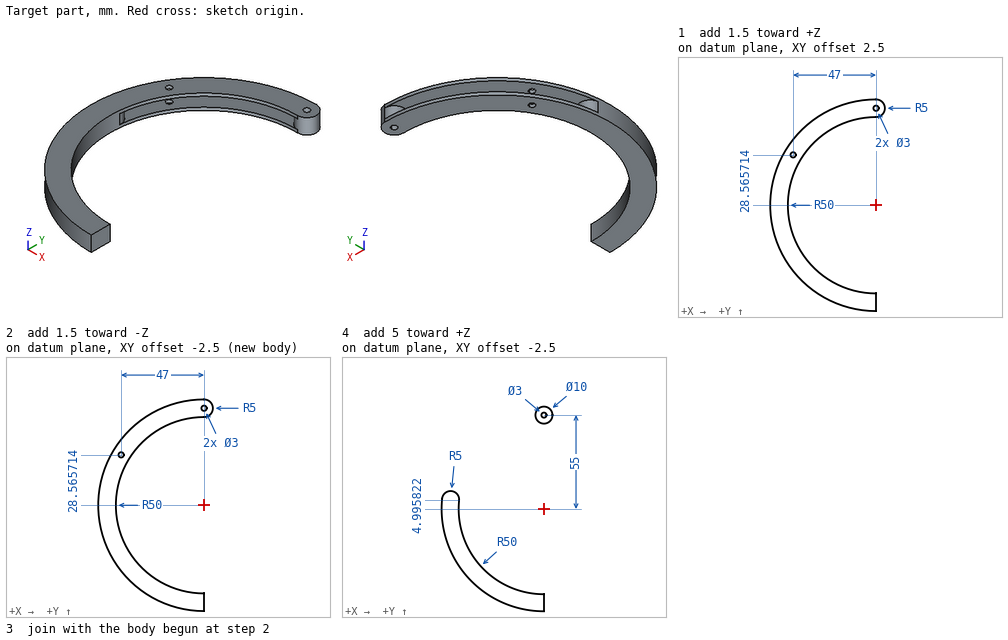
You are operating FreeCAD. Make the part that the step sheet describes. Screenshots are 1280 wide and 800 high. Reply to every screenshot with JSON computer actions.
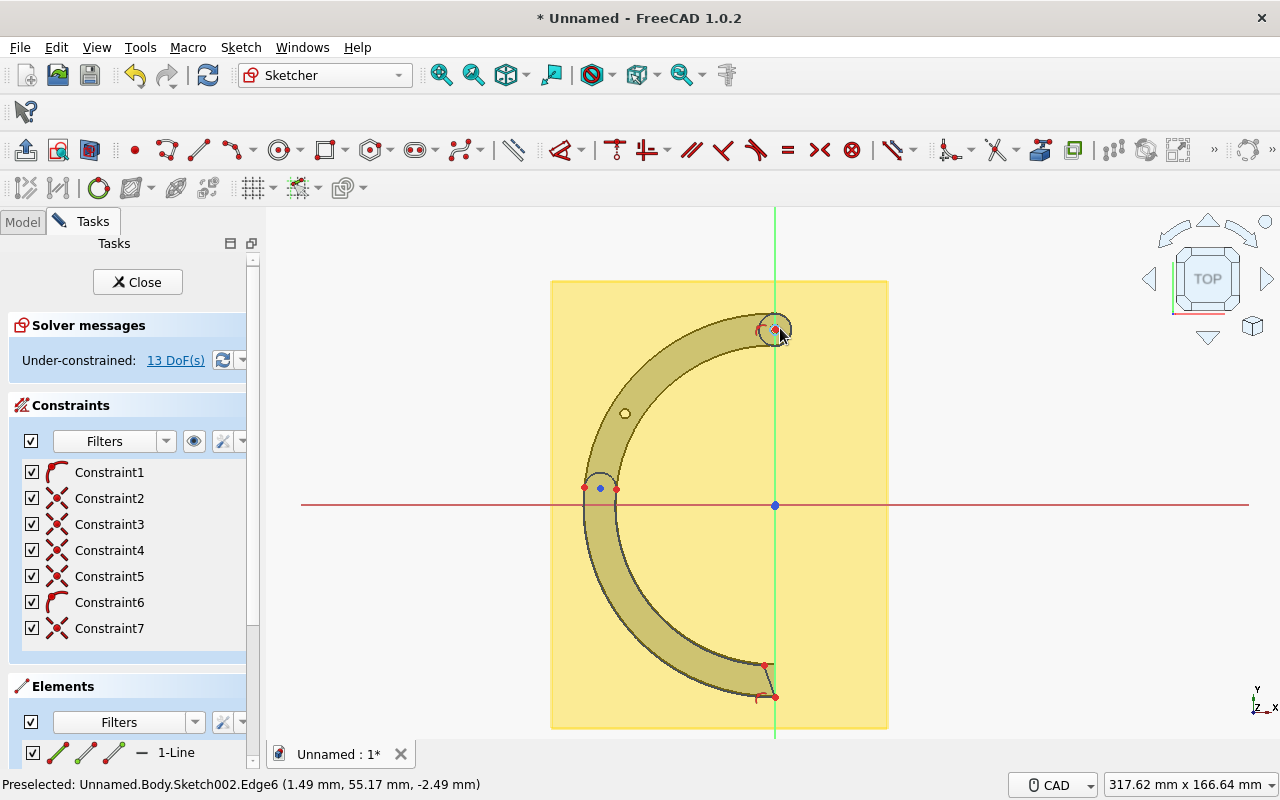
{"action": "left_click", "coordinate": [655, 522]}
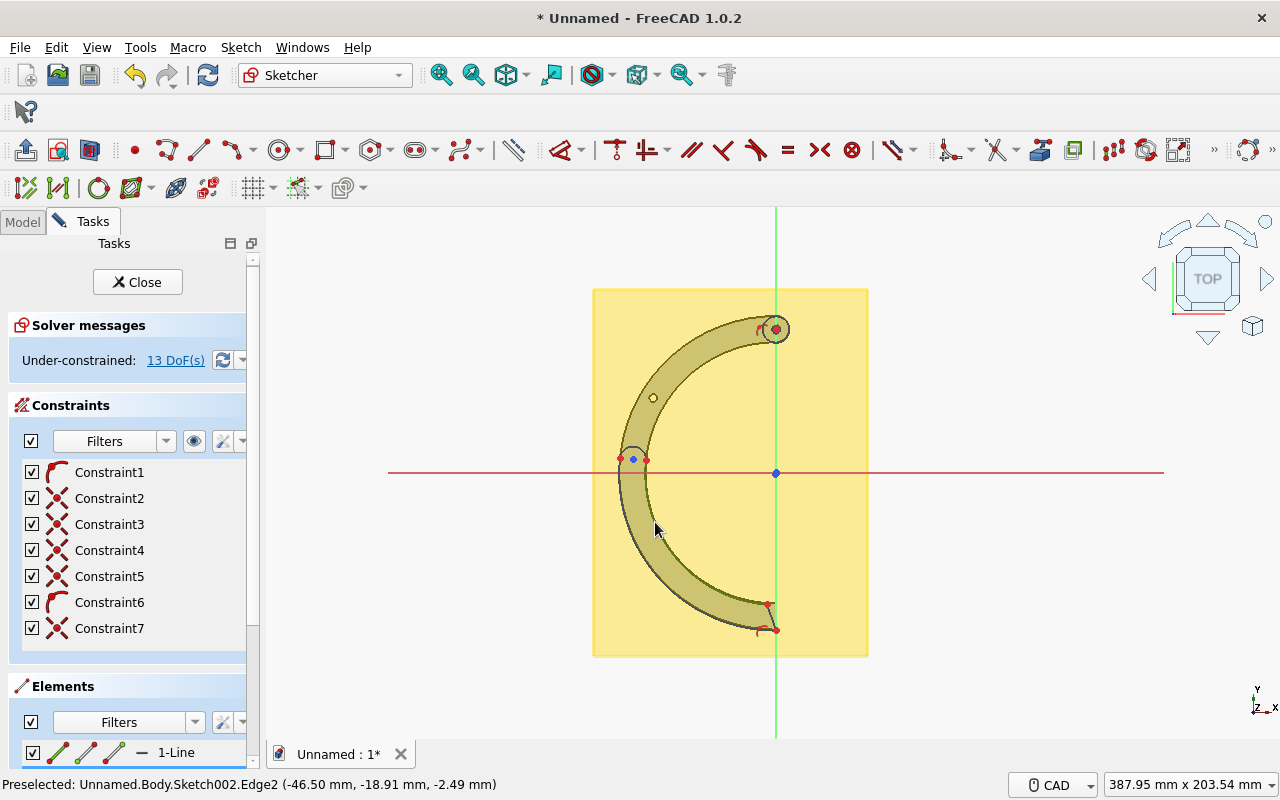
{"action": "left_click", "coordinate": [641, 450]}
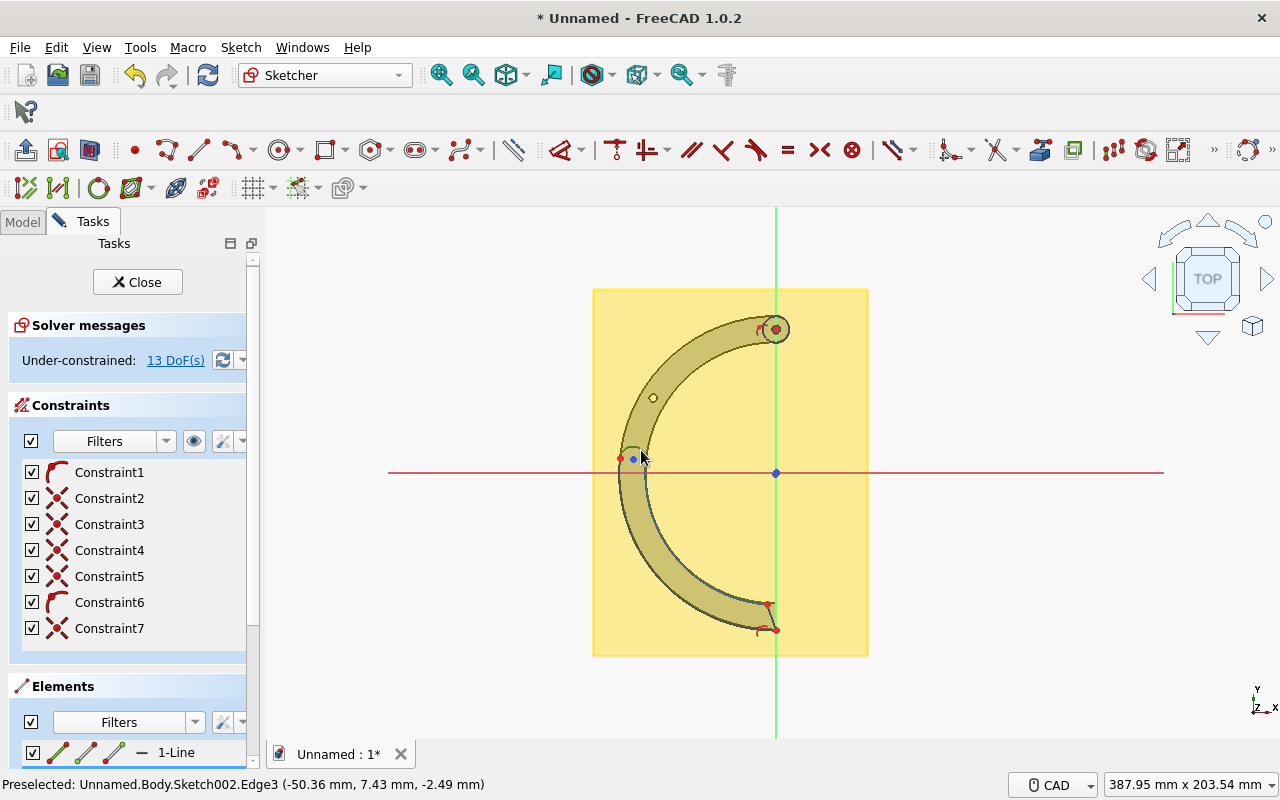
{"action": "left_click", "coordinate": [756, 150]}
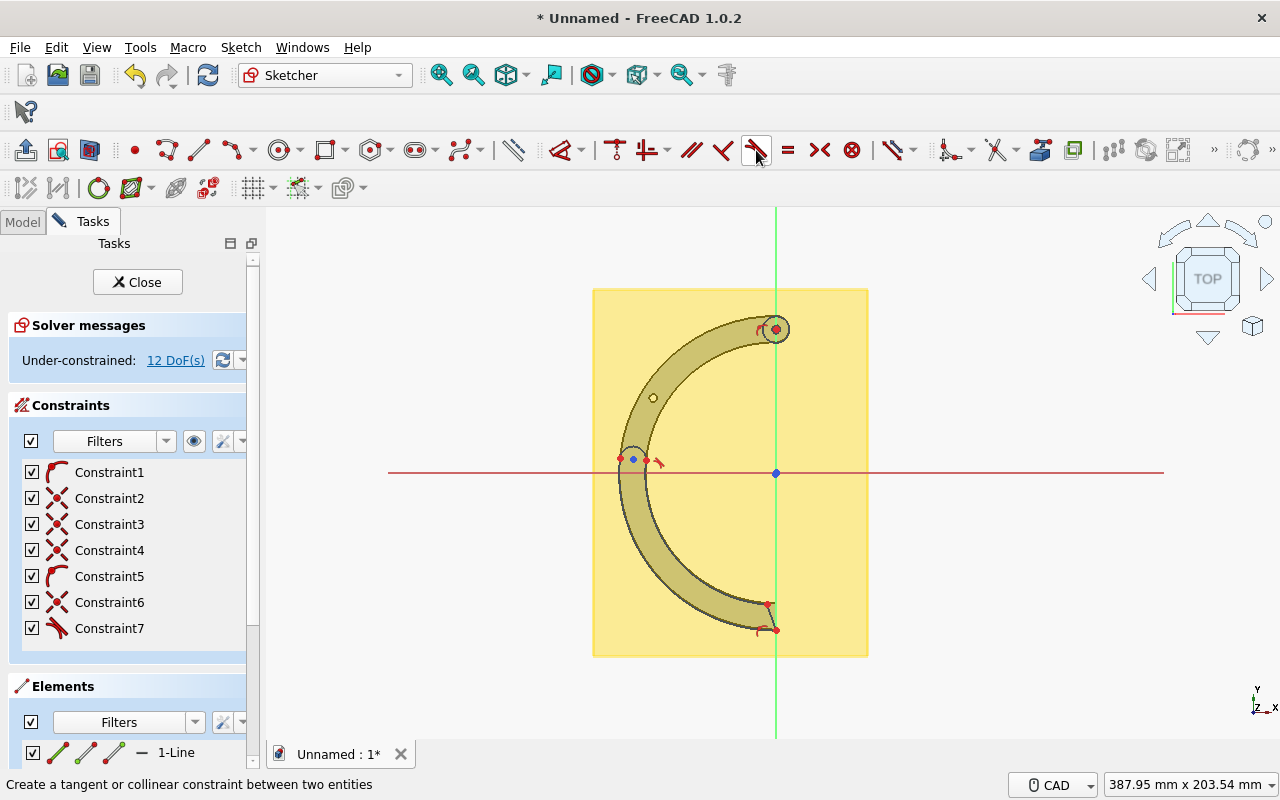
{"action": "left_click", "coordinate": [642, 450]}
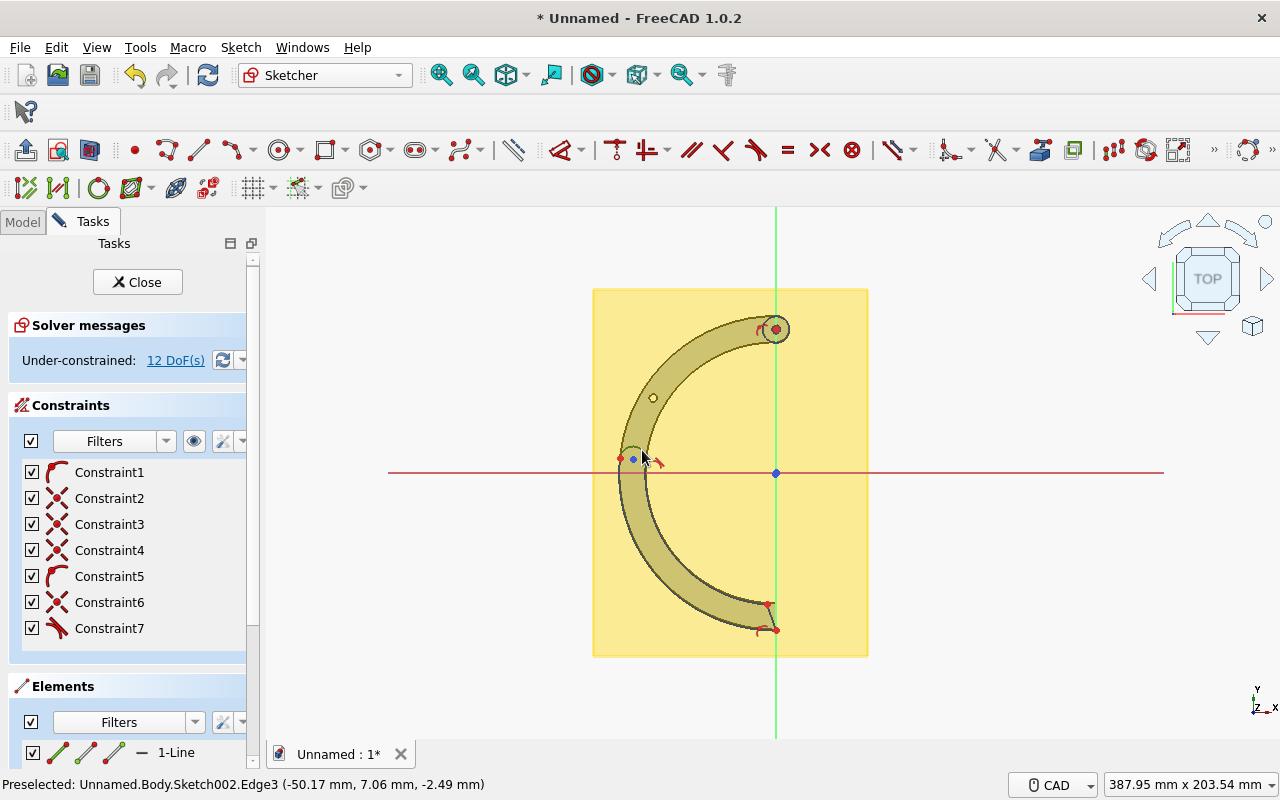
{"action": "left_click", "coordinate": [632, 535]}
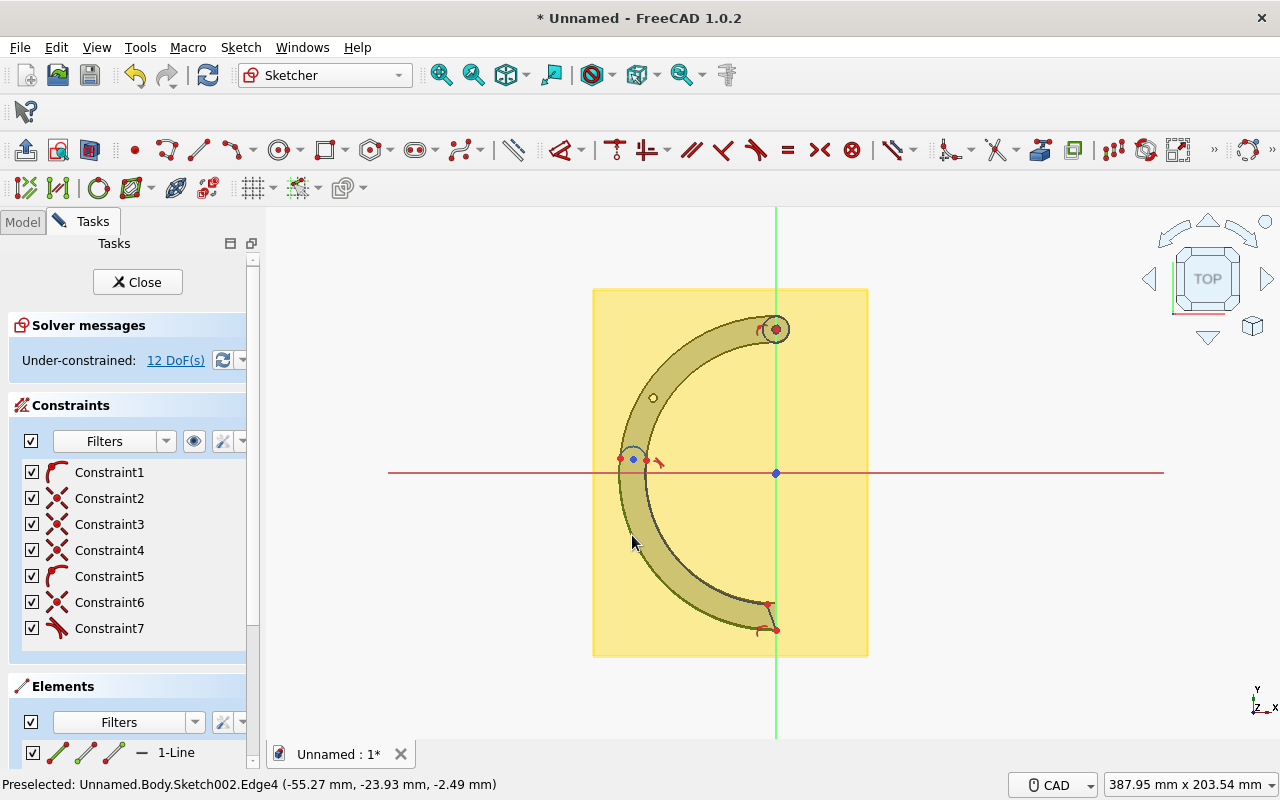
{"action": "left_click", "coordinate": [756, 150]}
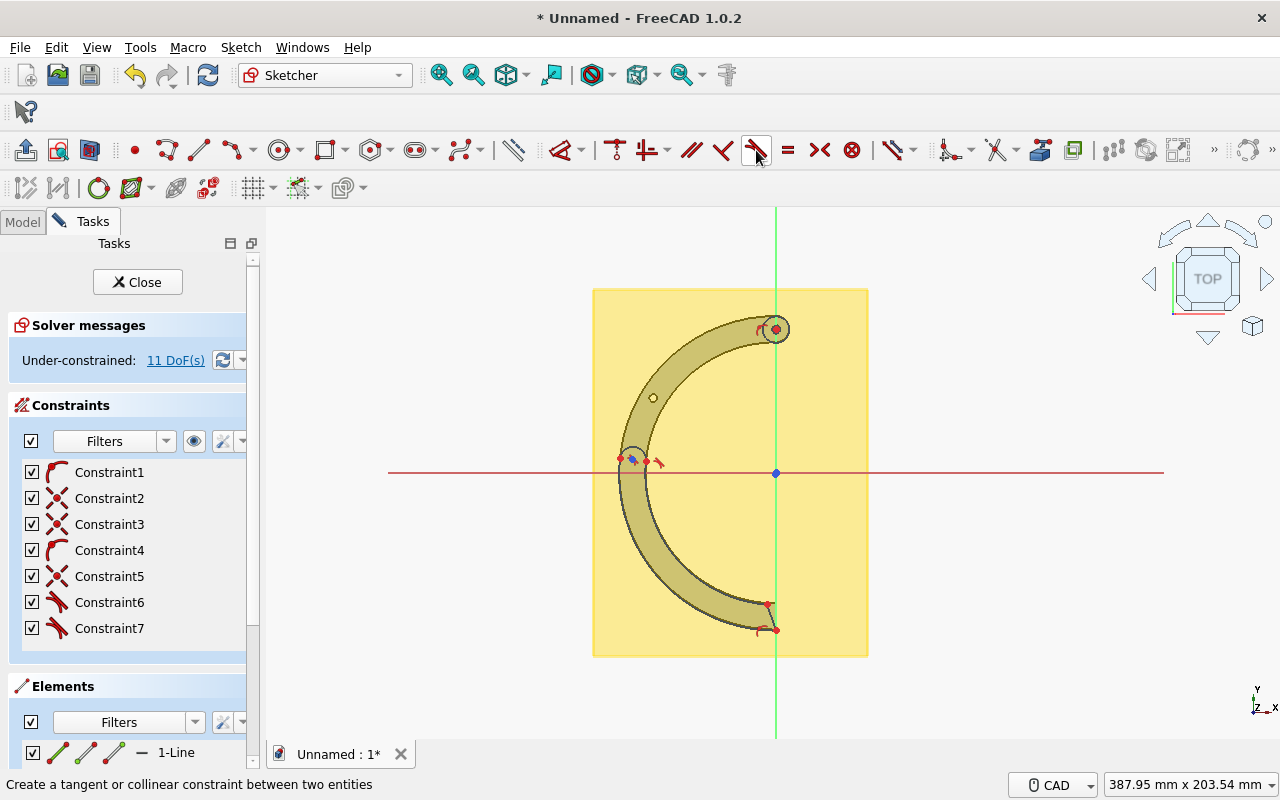
{"action": "scroll", "coordinate": [772, 620], "scroll_direction": "up", "scroll_amount": 2}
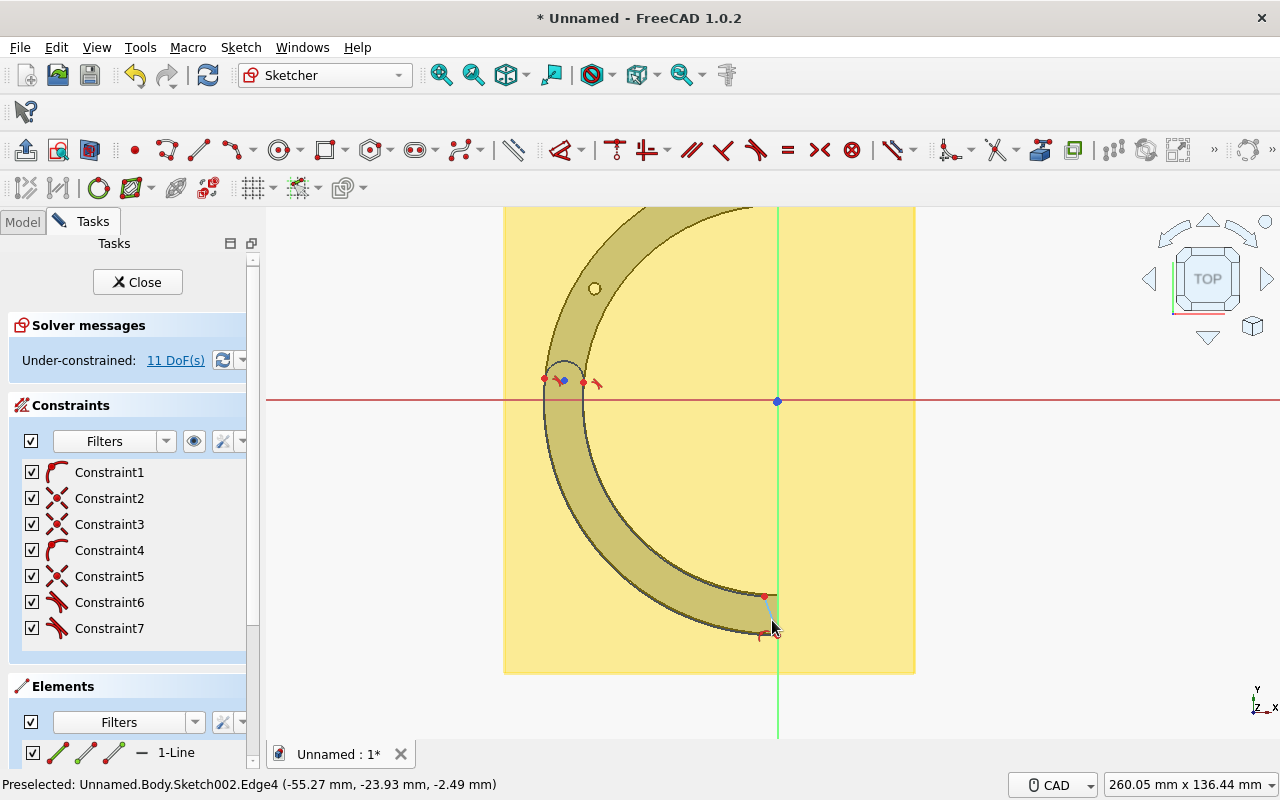
{"action": "left_click", "coordinate": [772, 620]}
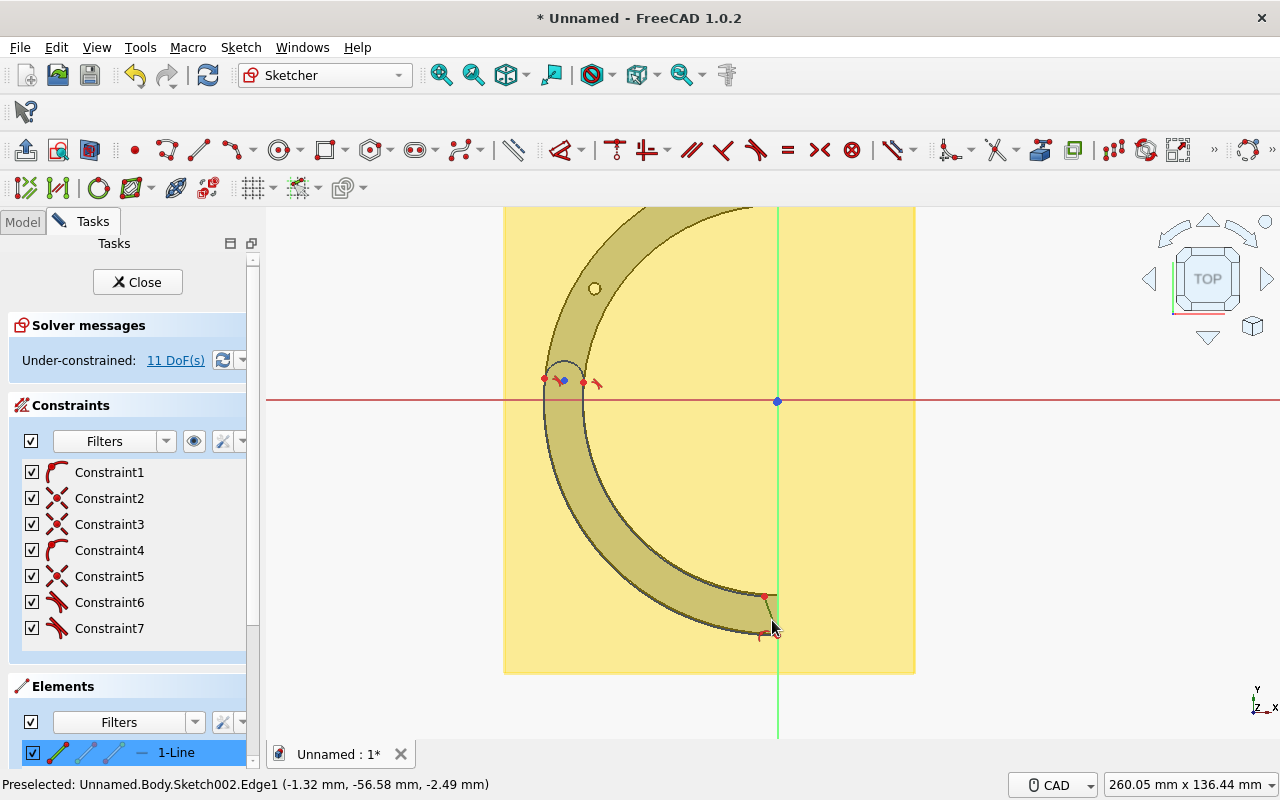
{"action": "left_click", "coordinate": [670, 150]}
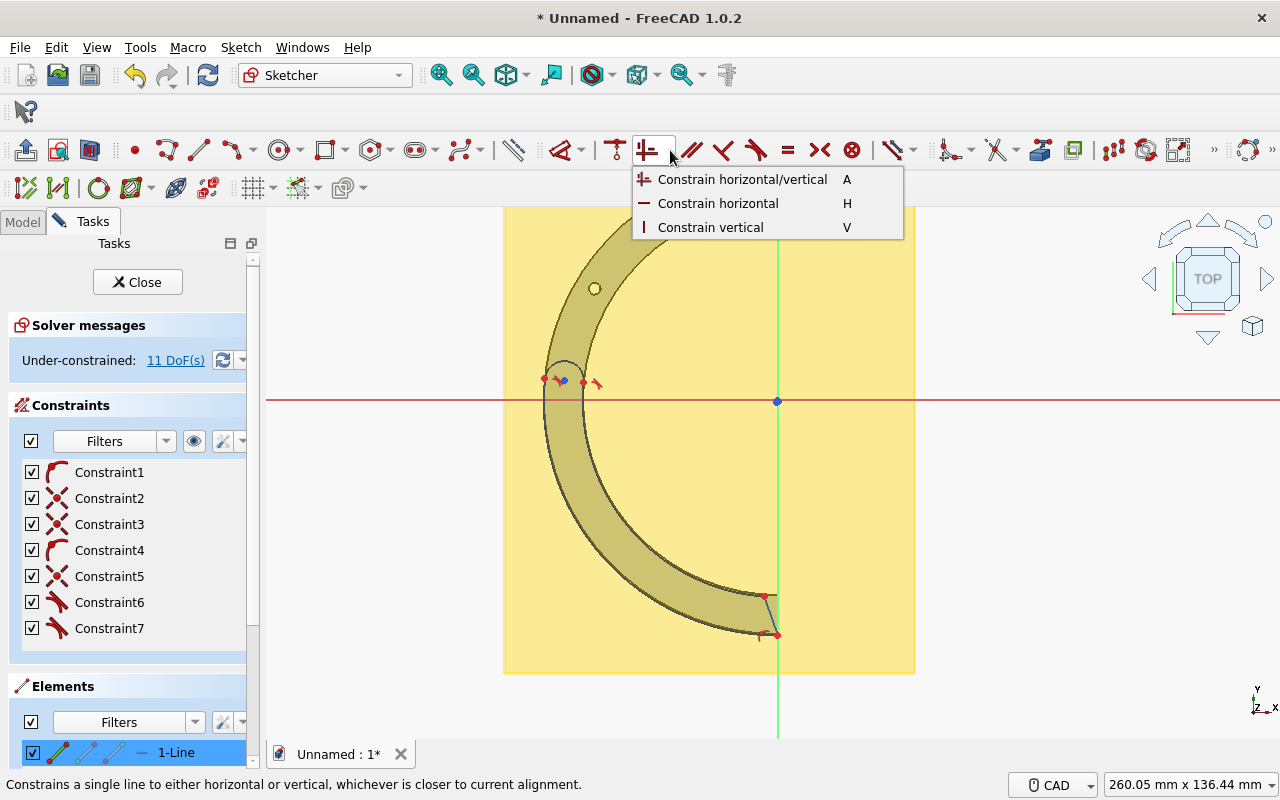
{"action": "left_click", "coordinate": [768, 227]}